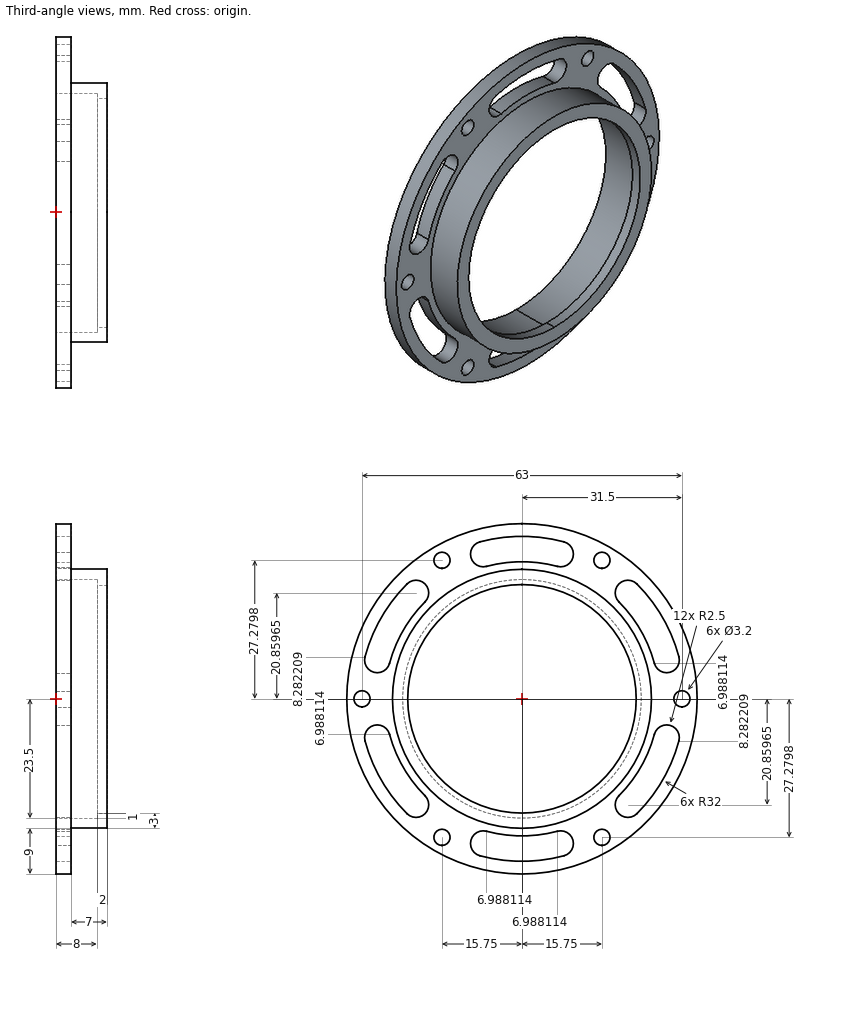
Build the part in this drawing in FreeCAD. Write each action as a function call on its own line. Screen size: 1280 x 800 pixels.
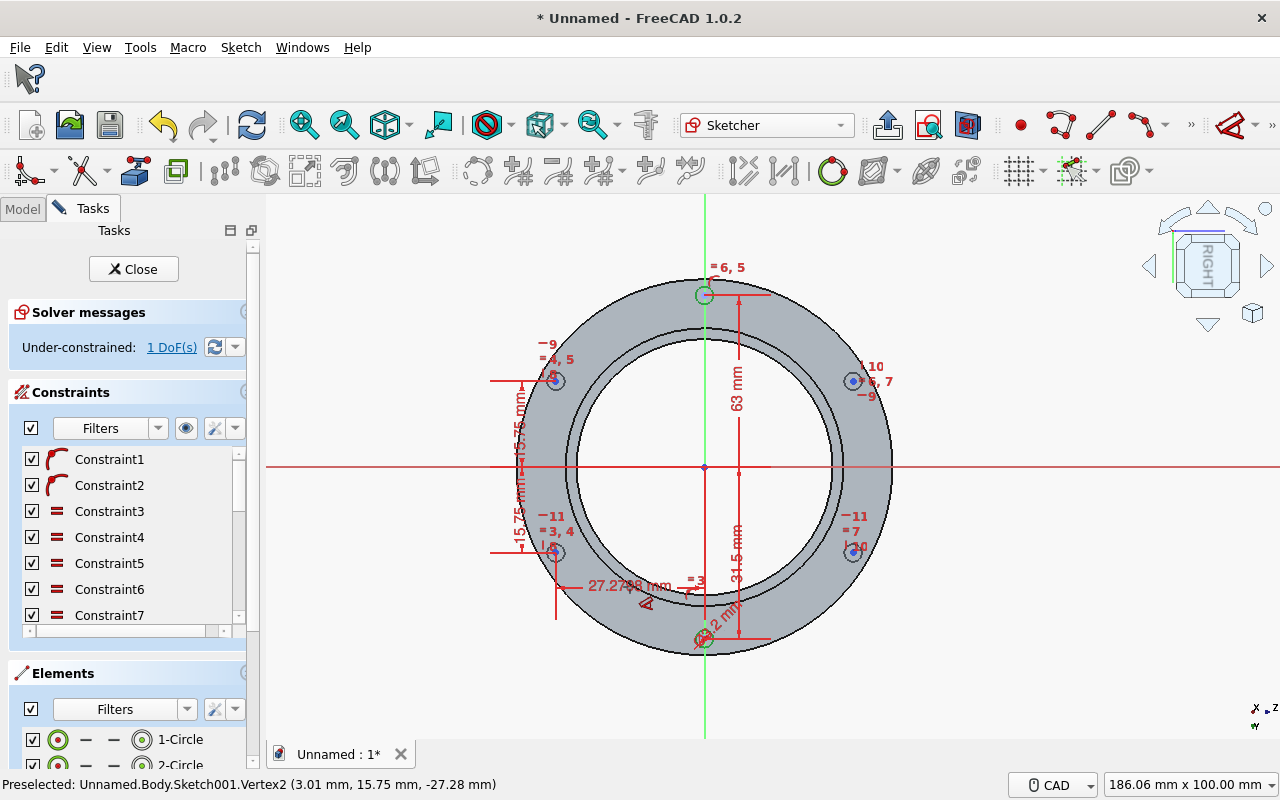
click(853, 381)
click(779, 347)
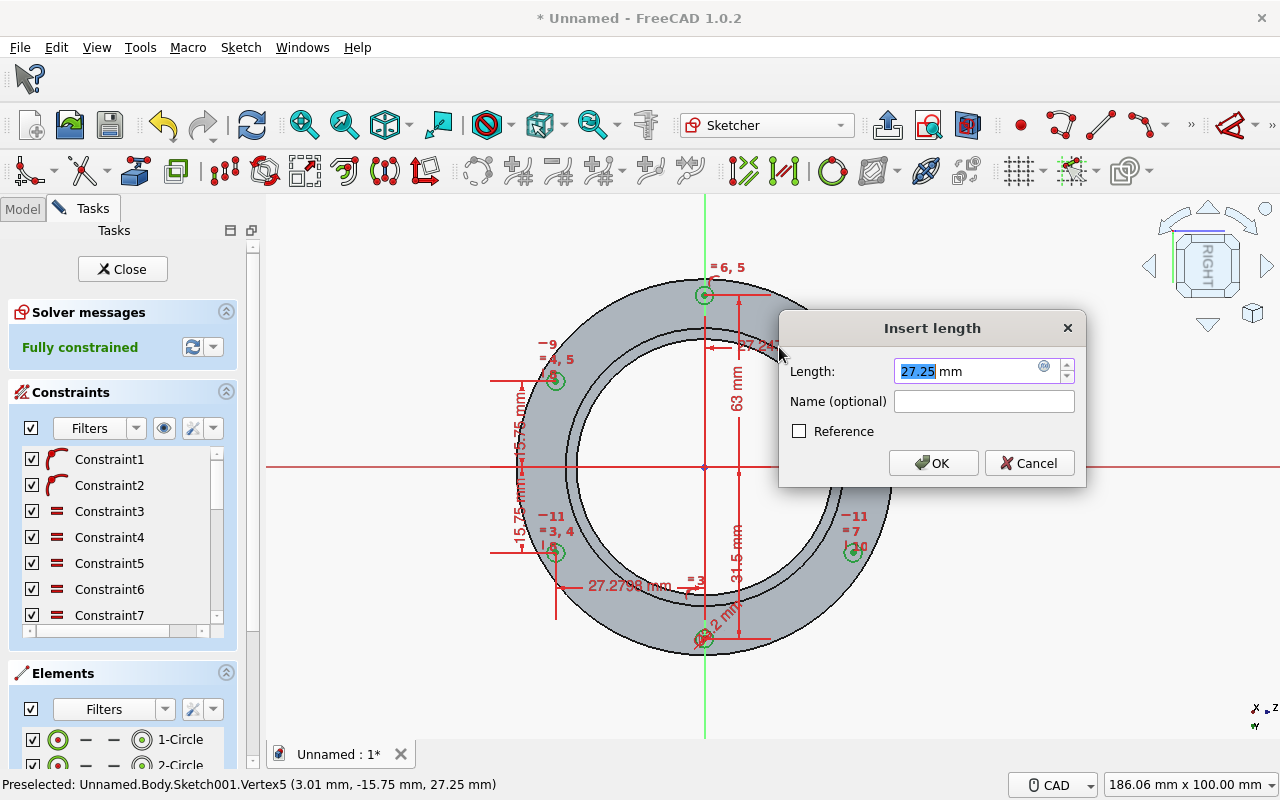
text(27.2798)
key(Return)
key(Escape)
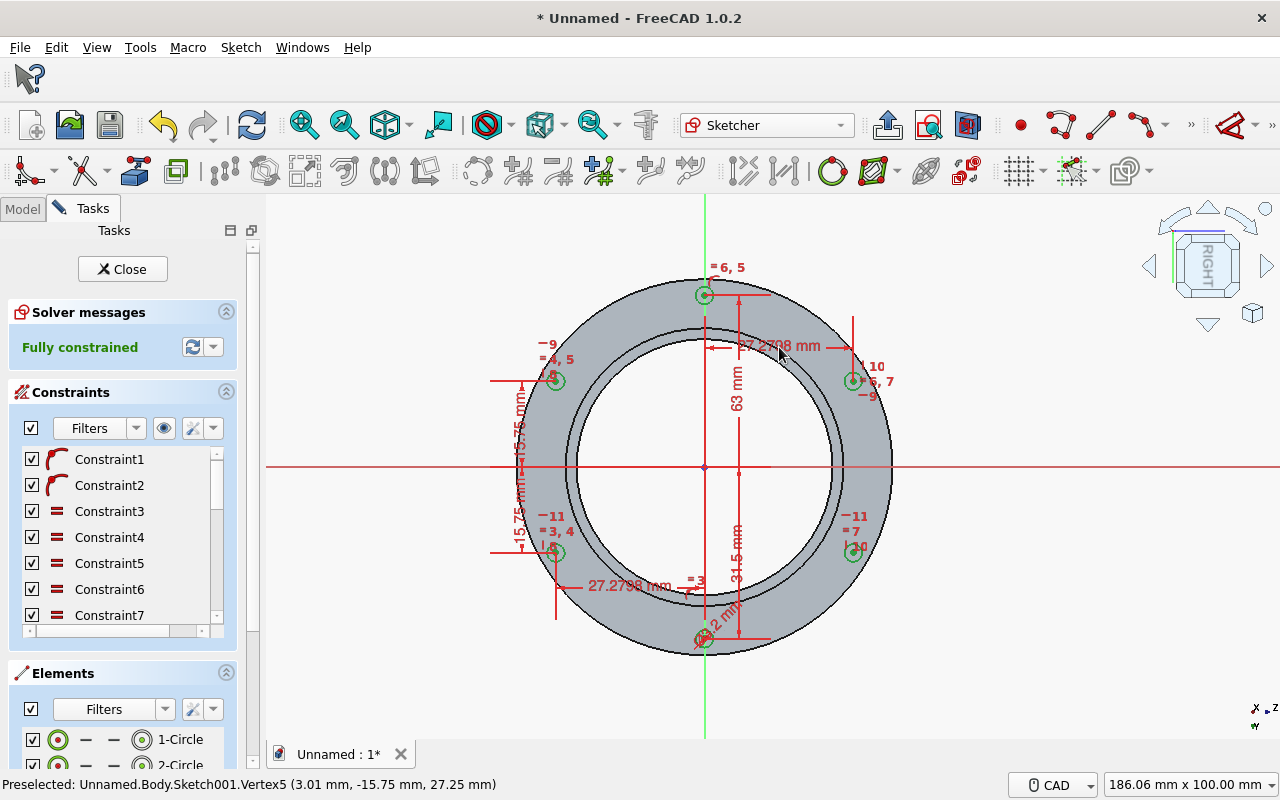
click(123, 269)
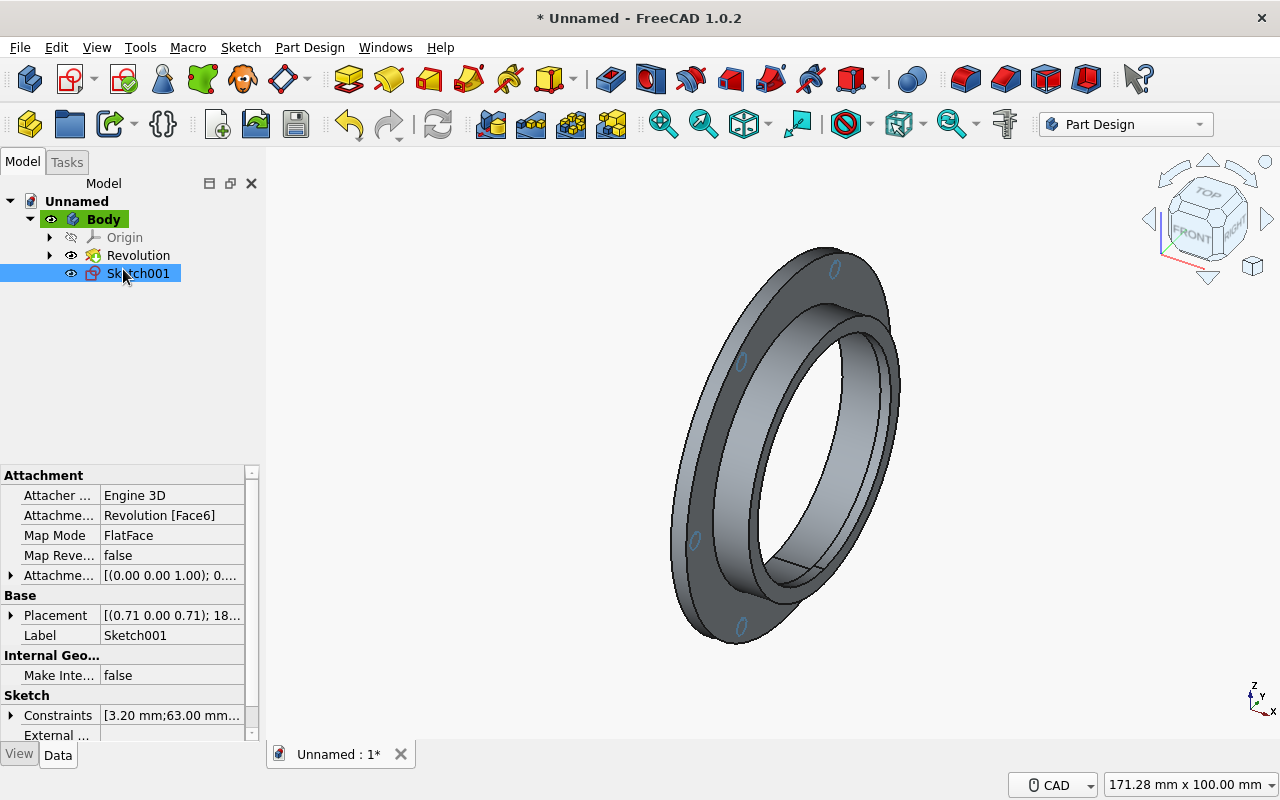
click(612, 80)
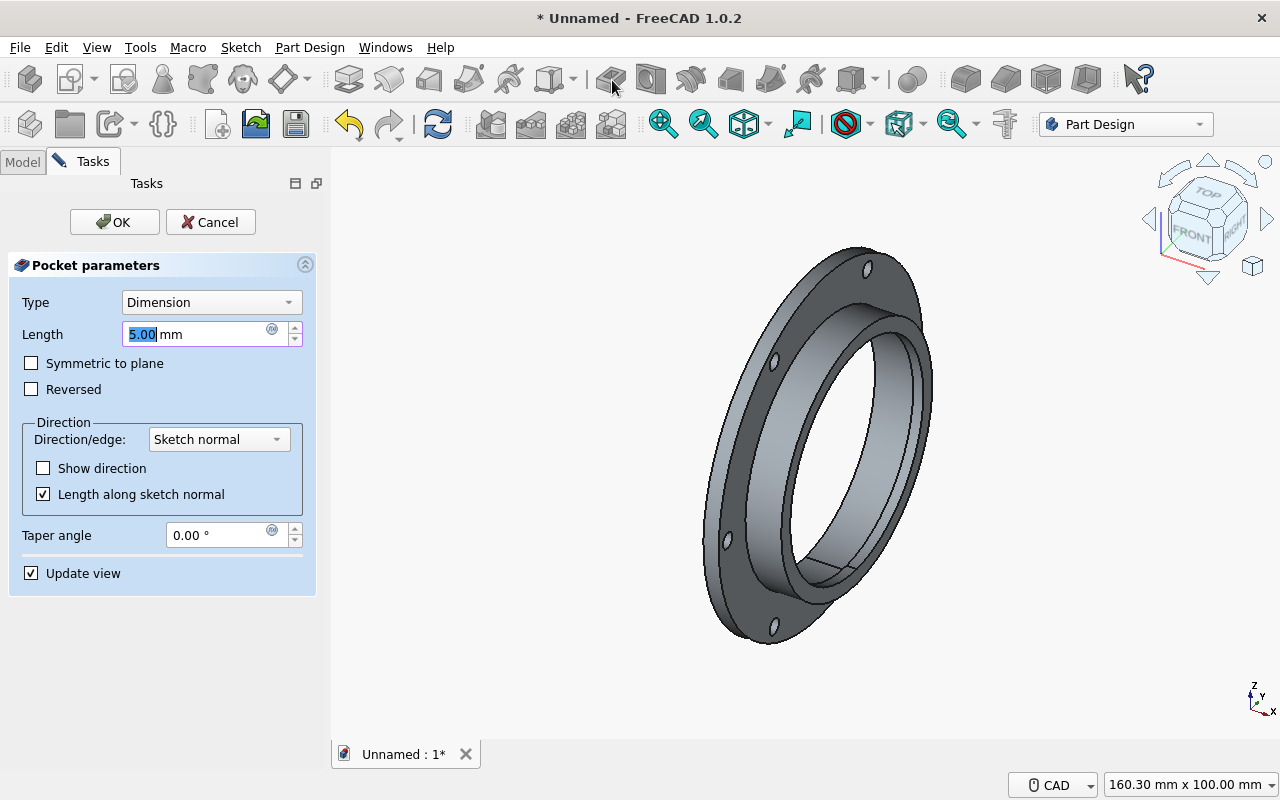
click(212, 302)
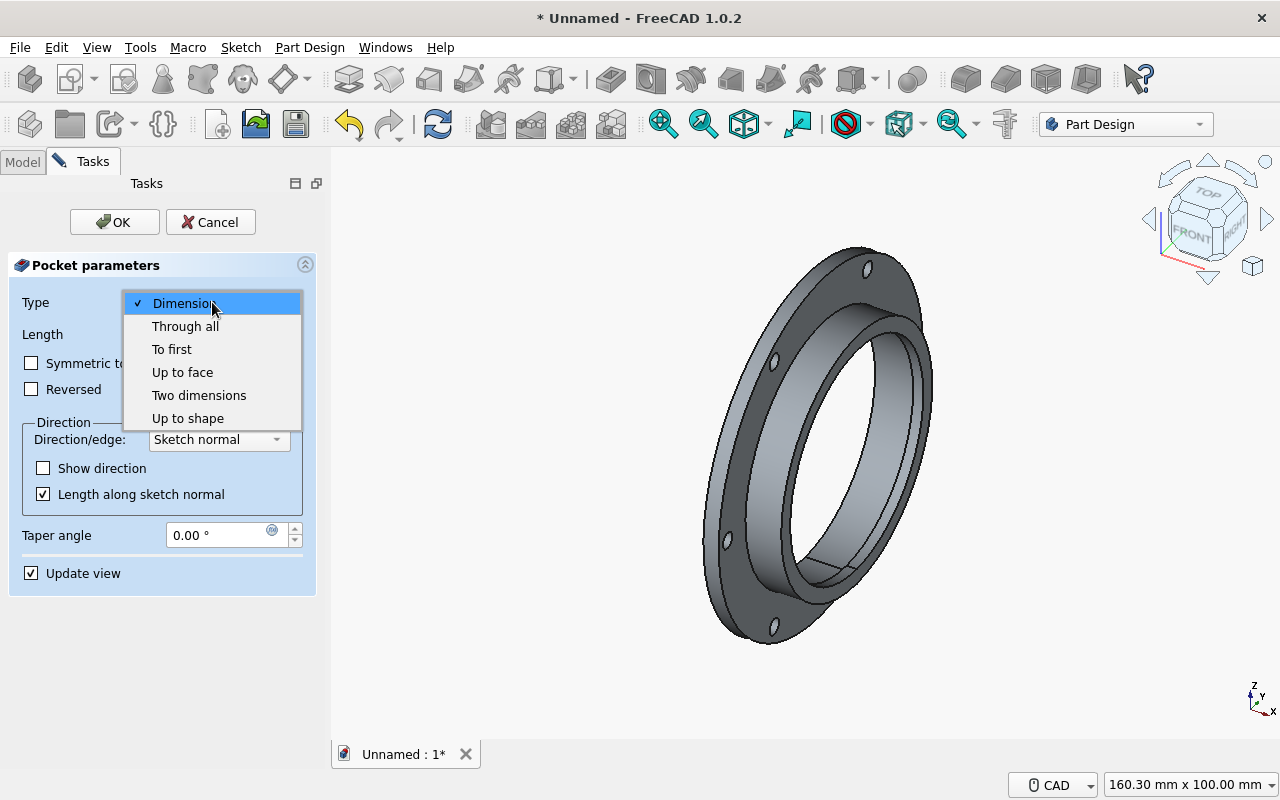
click(212, 326)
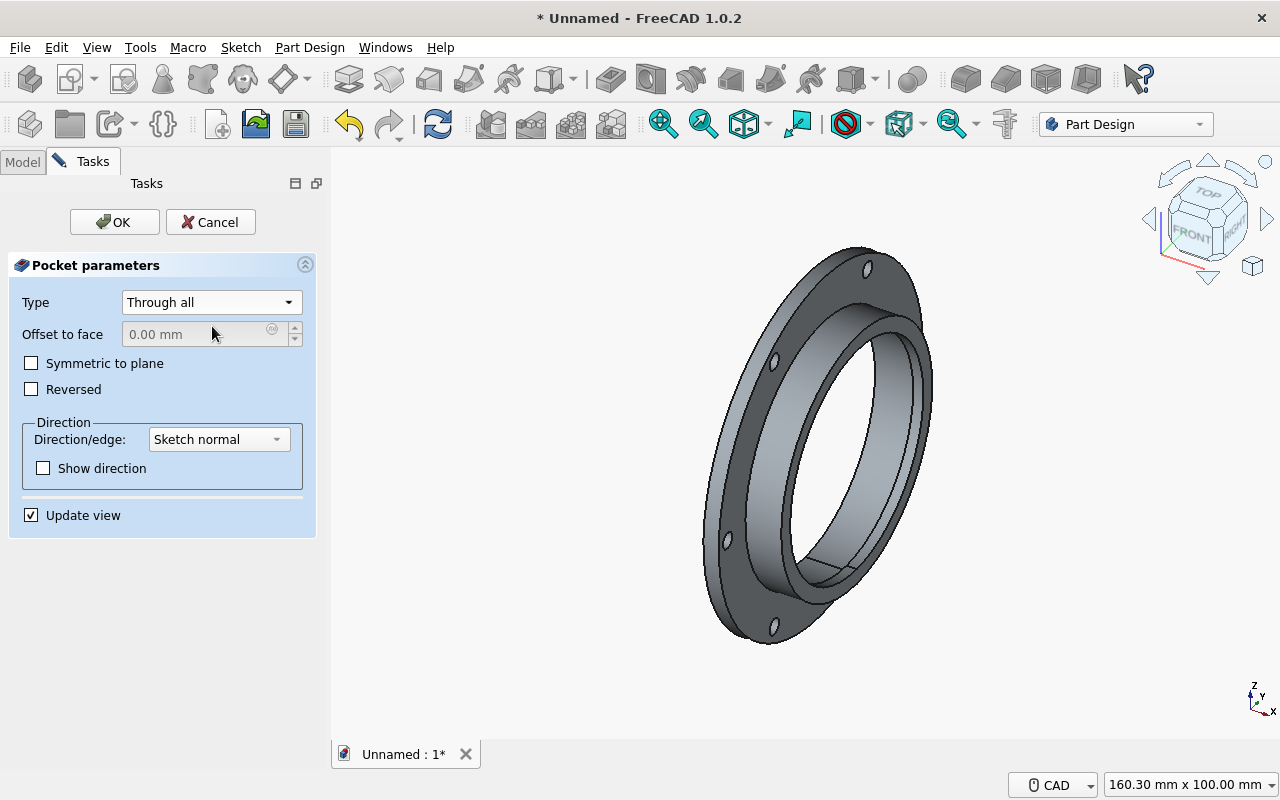
click(115, 222)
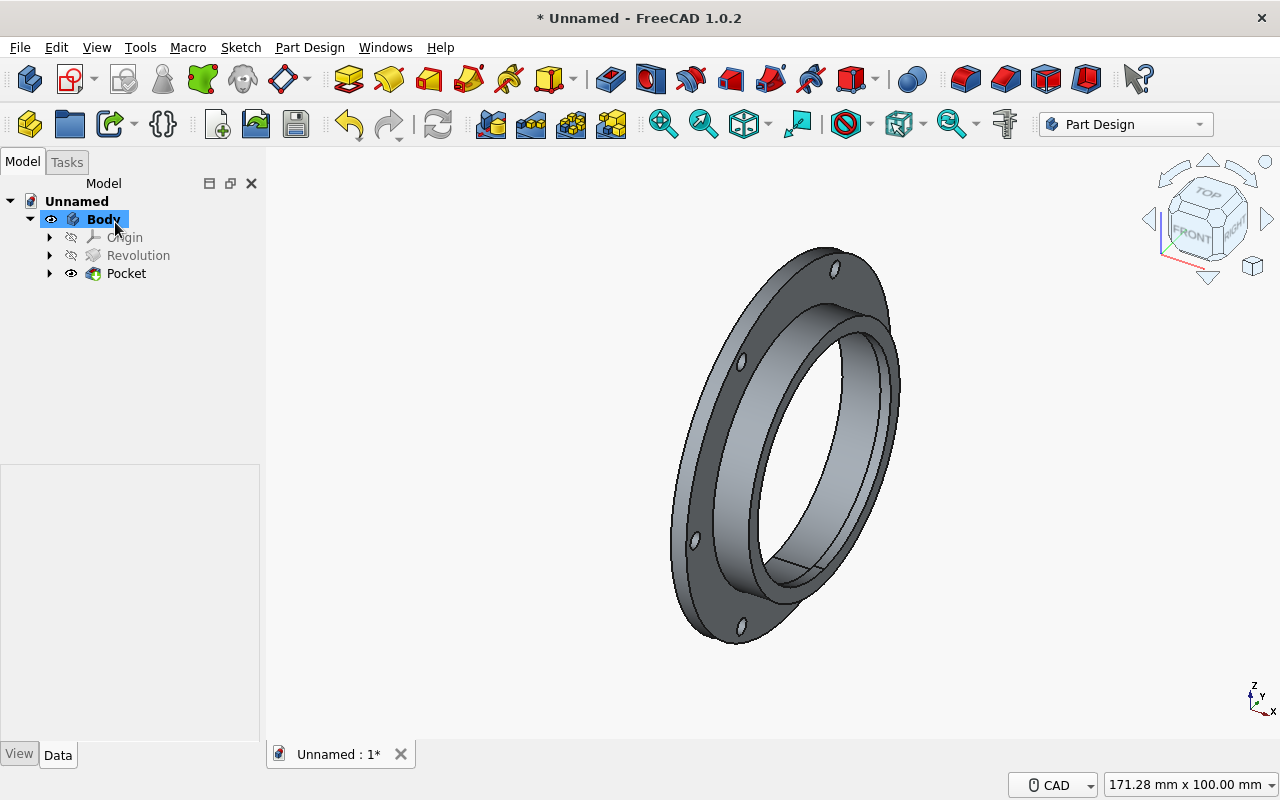
click(788, 304)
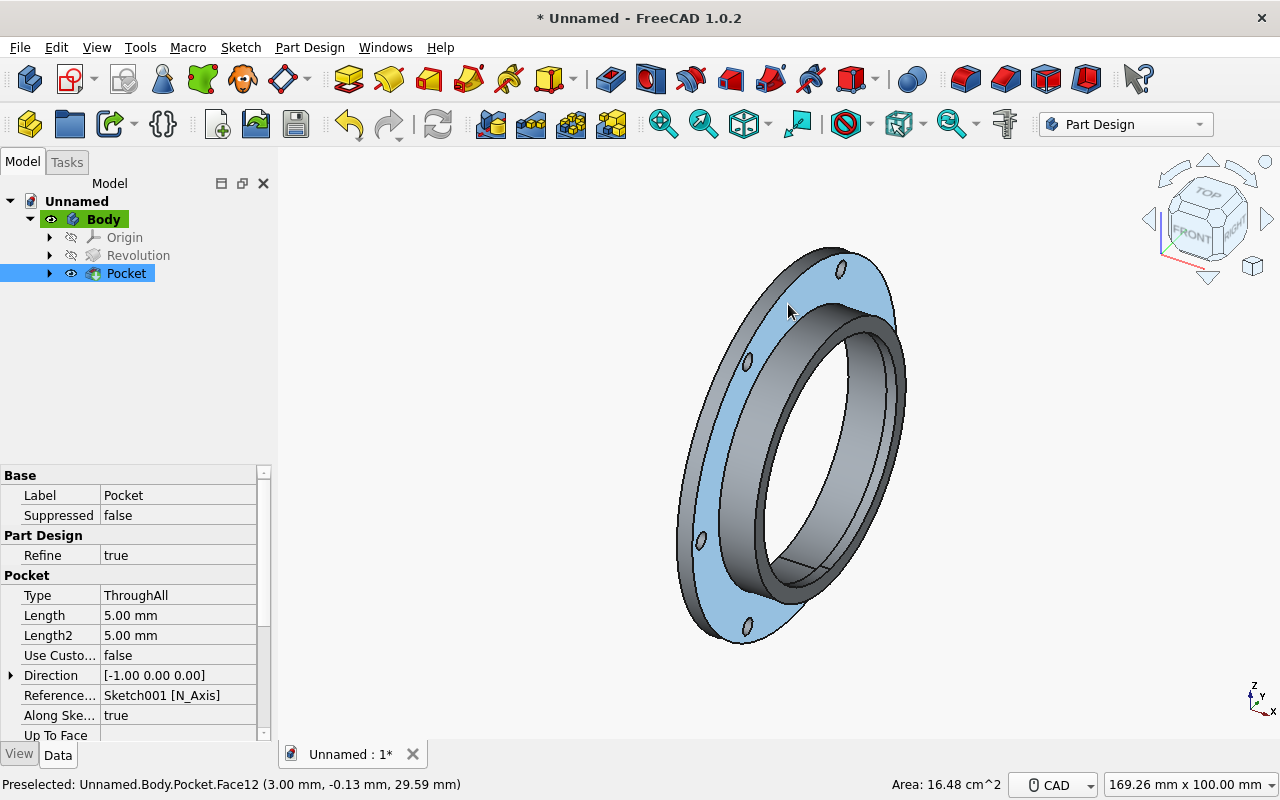
click(70, 80)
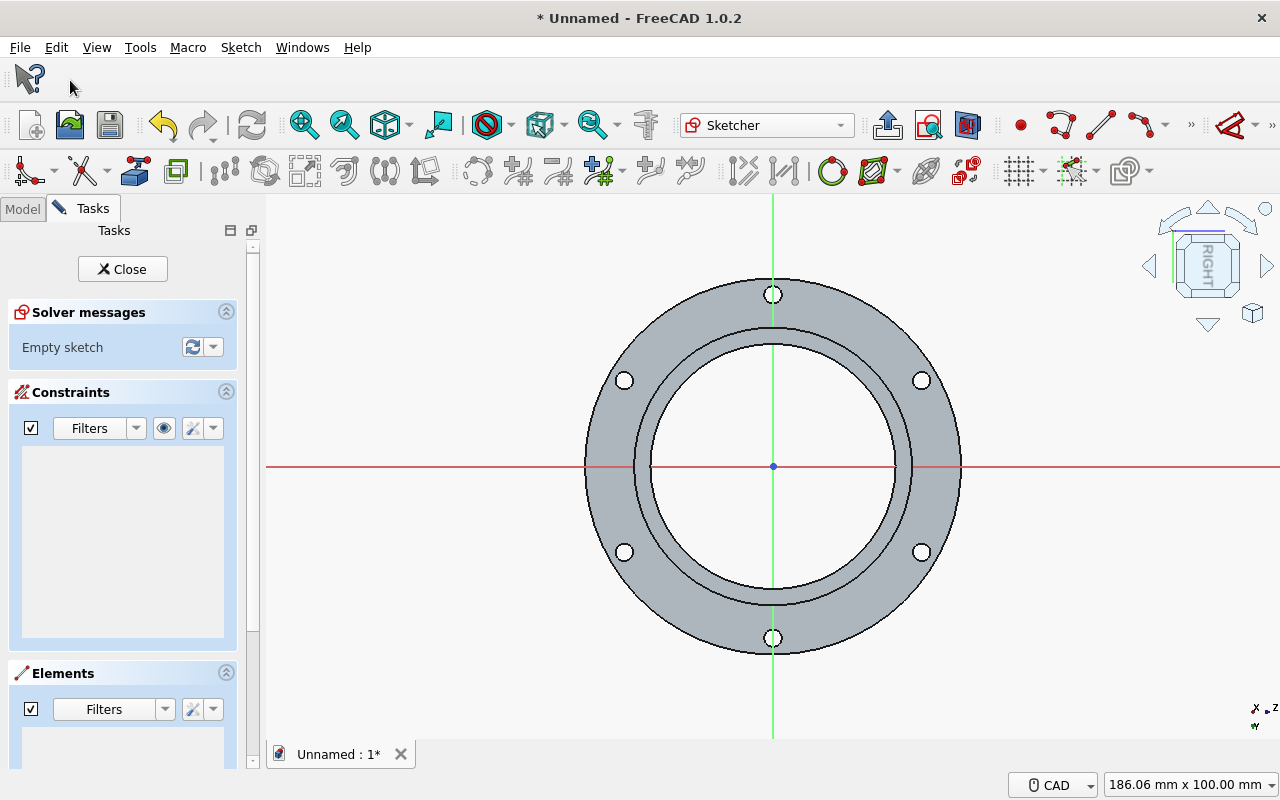
key(g)
key(3)
key(a)